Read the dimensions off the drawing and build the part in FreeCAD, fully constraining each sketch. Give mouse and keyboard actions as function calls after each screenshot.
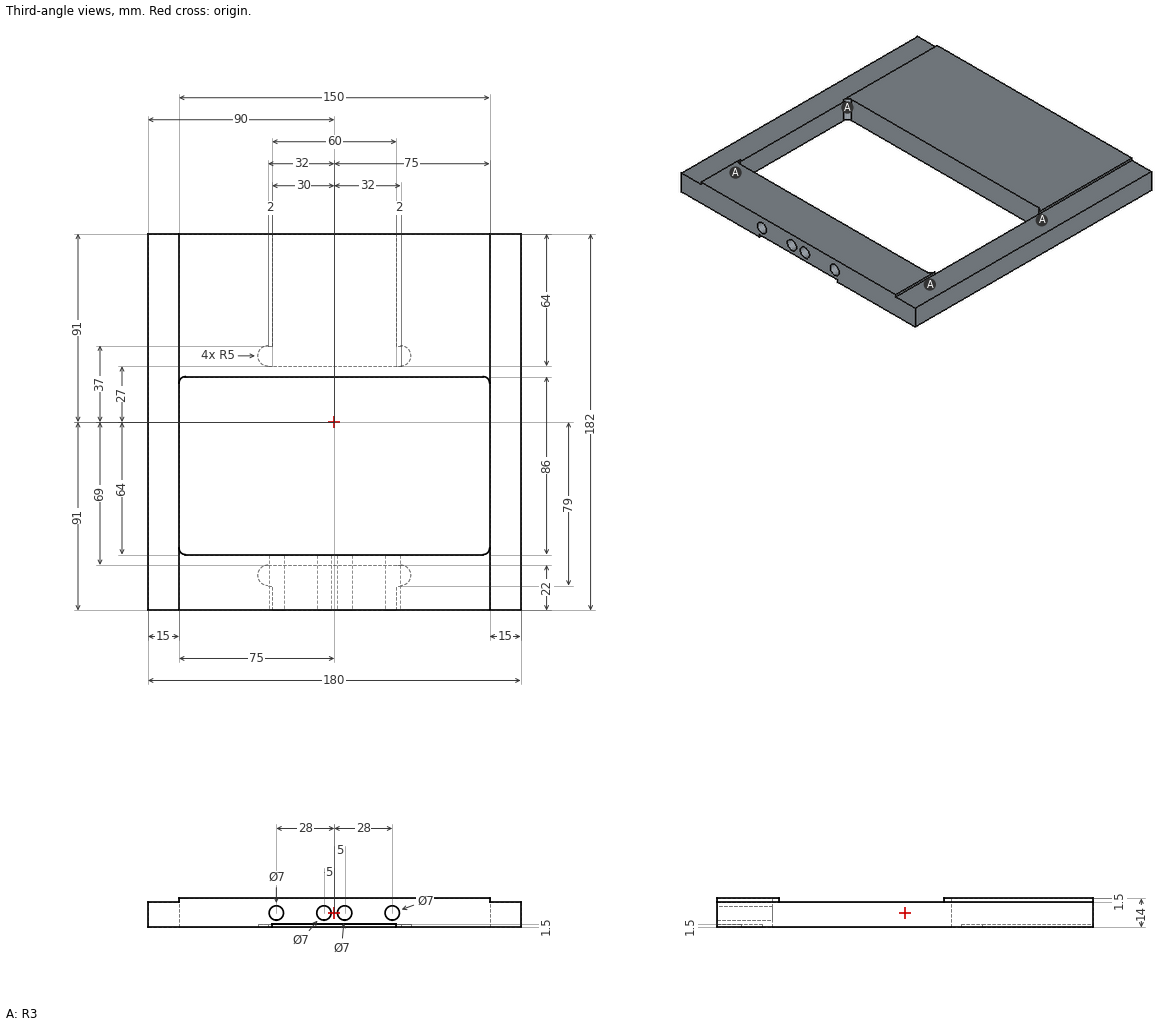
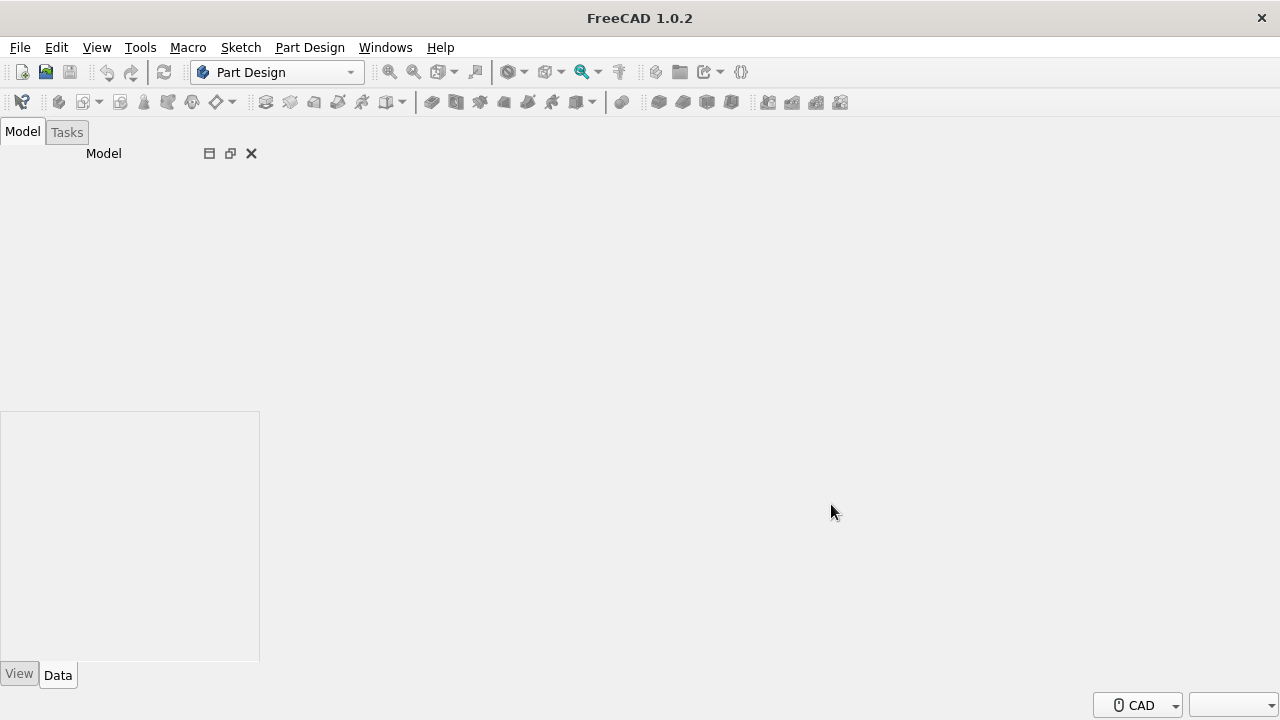
key(ctrl+n)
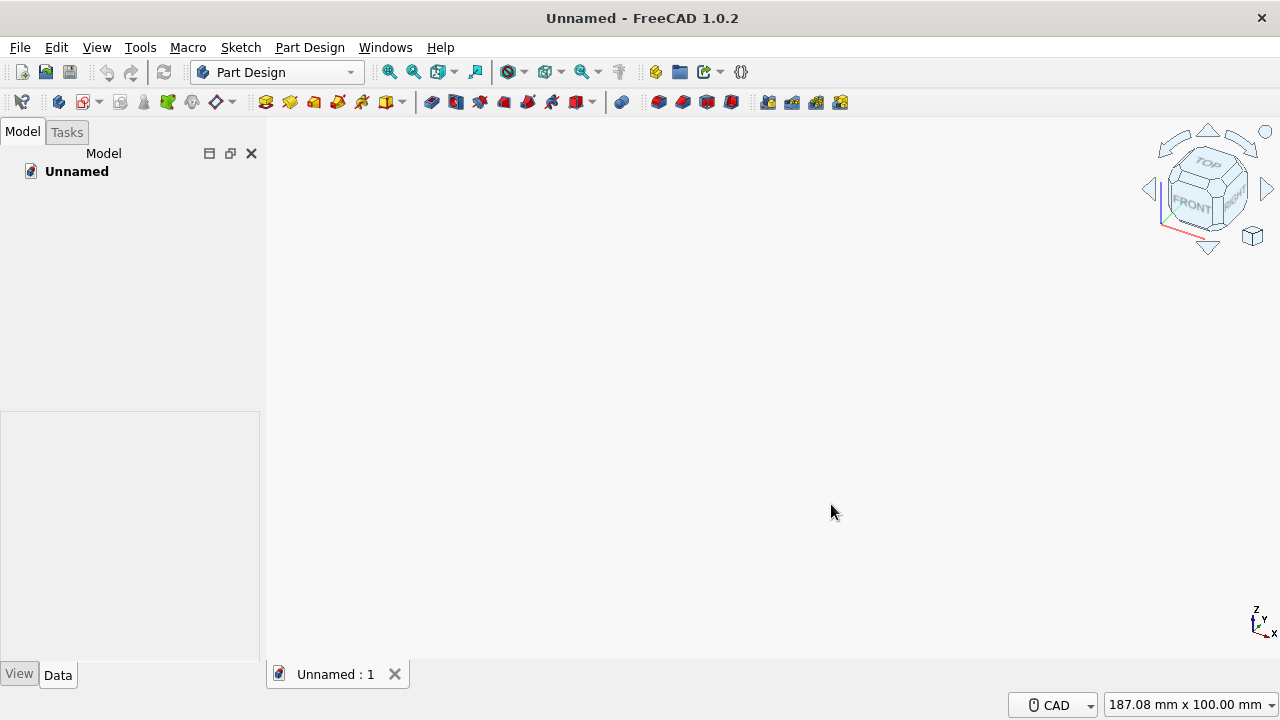
click(84, 102)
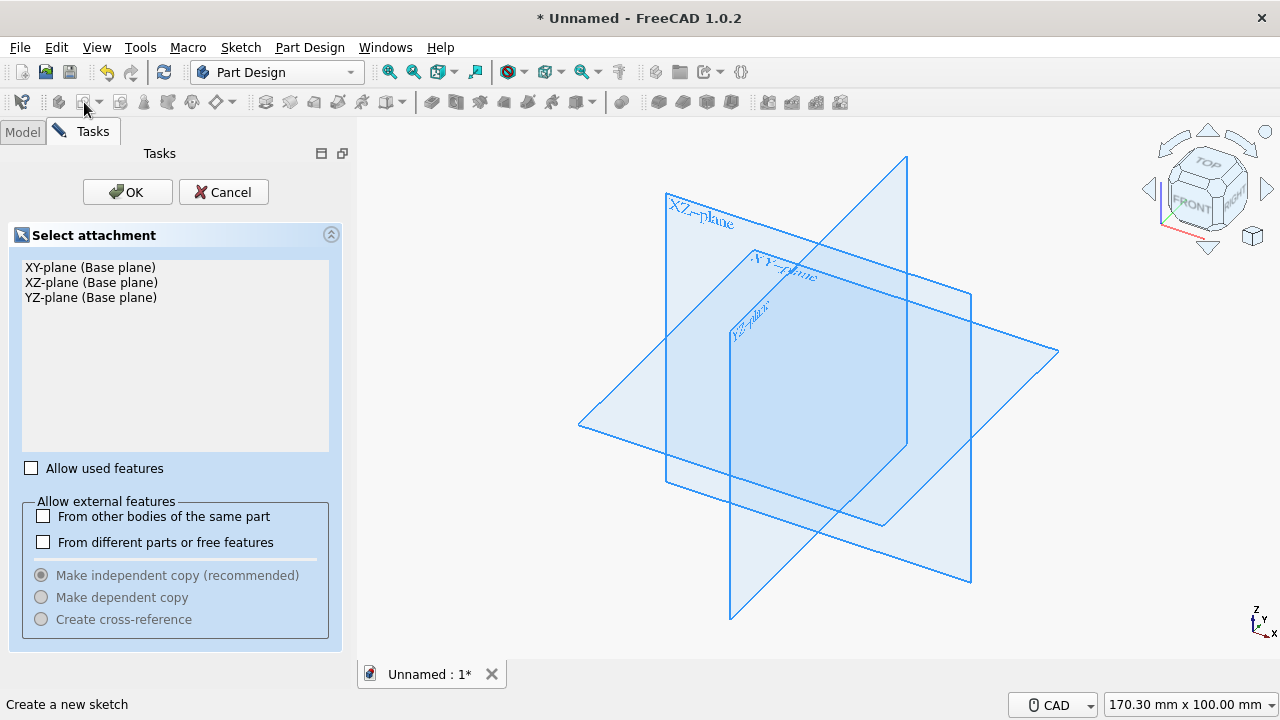
click(82, 268)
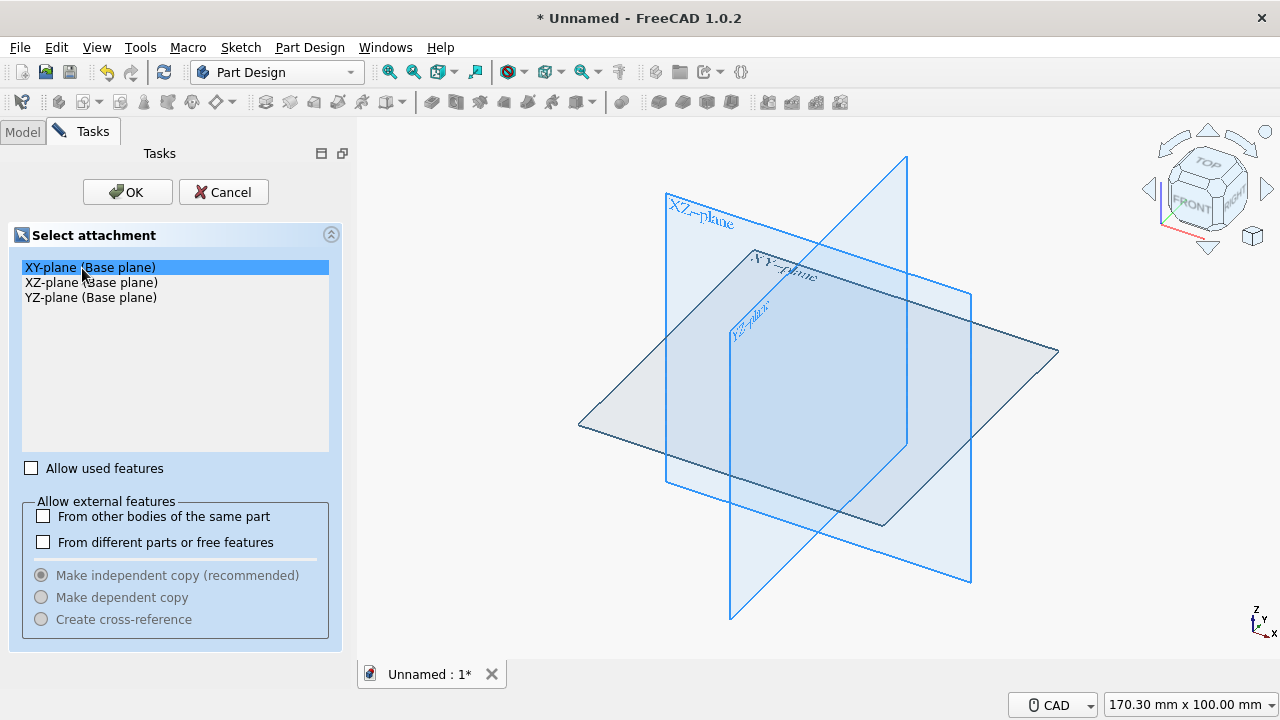
click(128, 192)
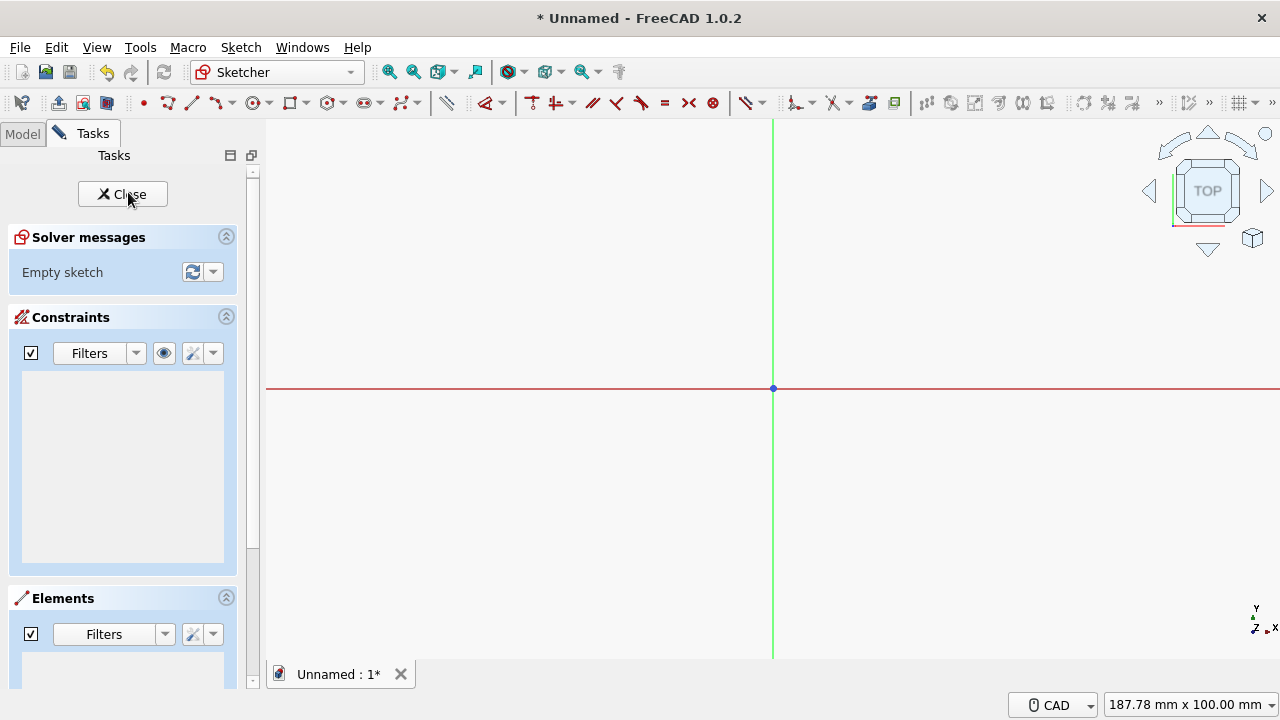
scroll(665, 389, down, 5)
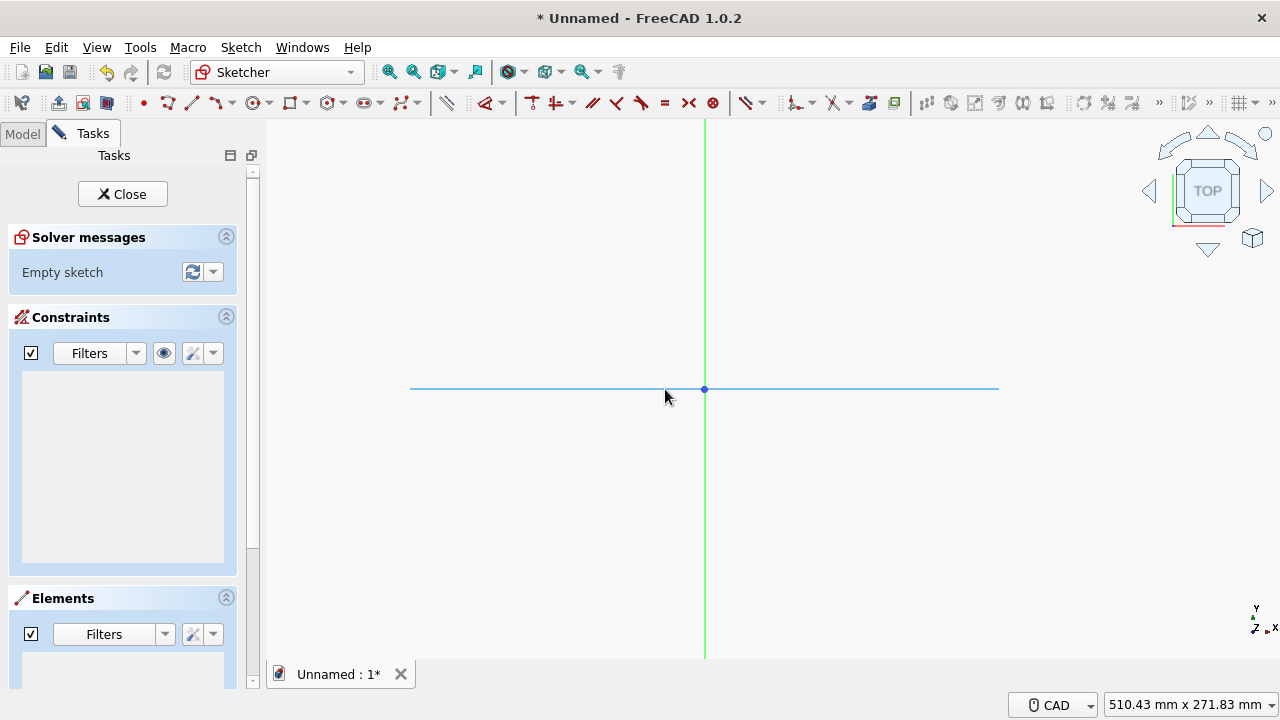
click(308, 104)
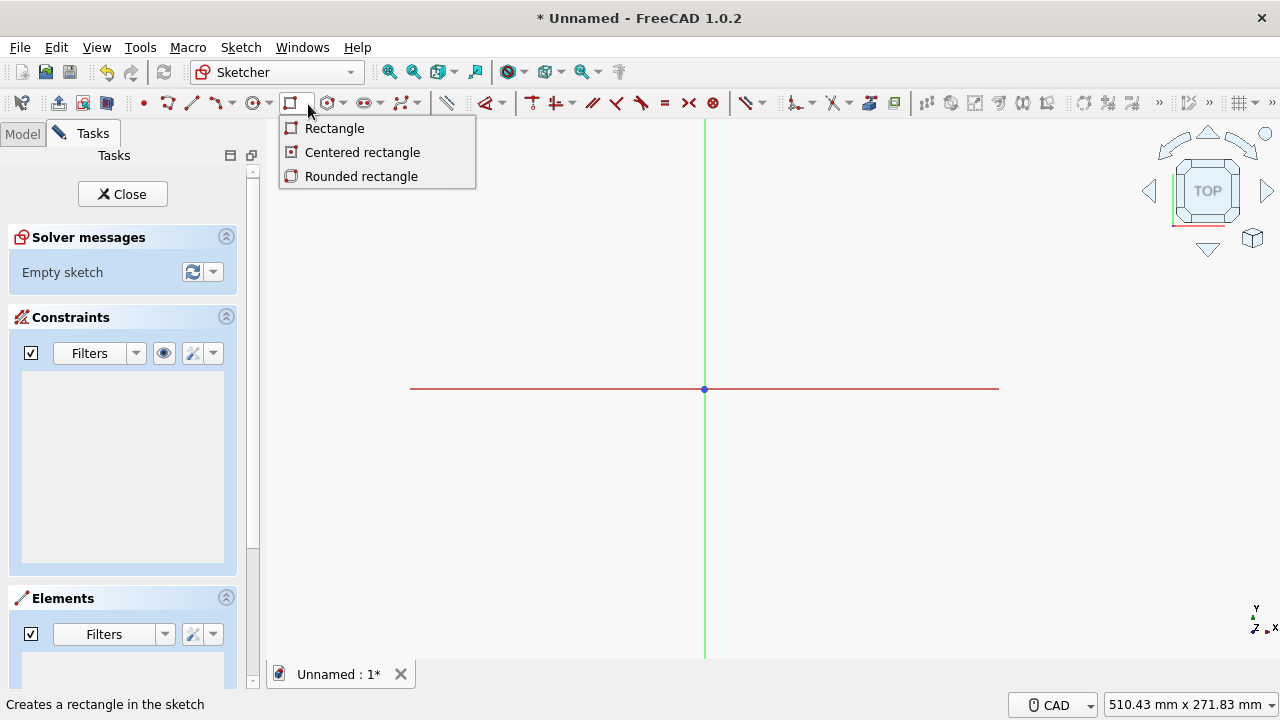
click(378, 152)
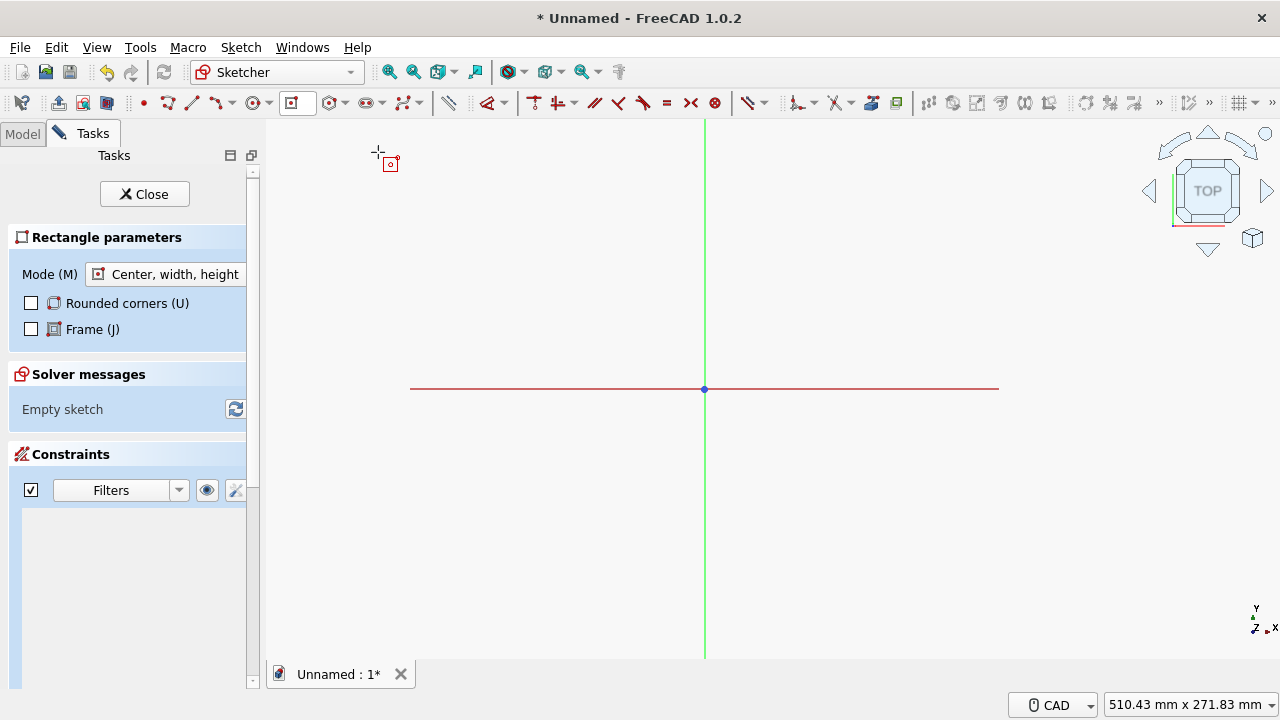
click(705, 389)
move(884, 209)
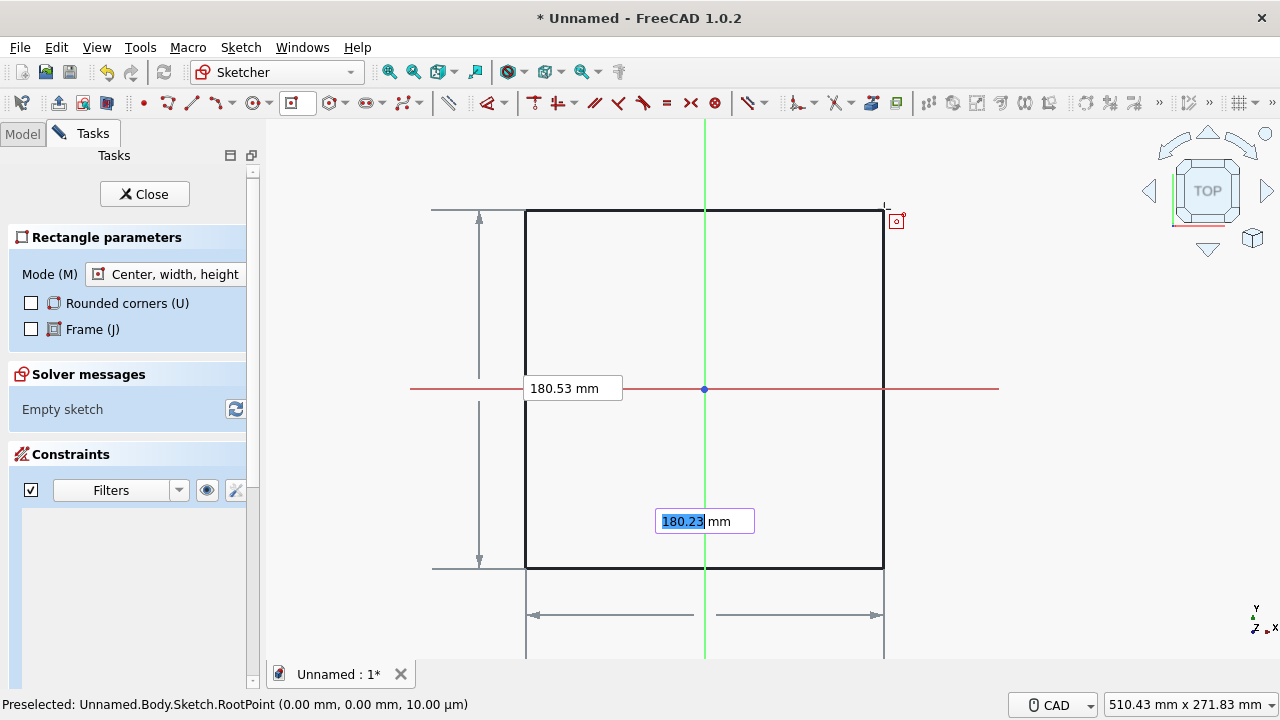
text(180)
key(Tab)
text(182)
key(Return)
key(Escape)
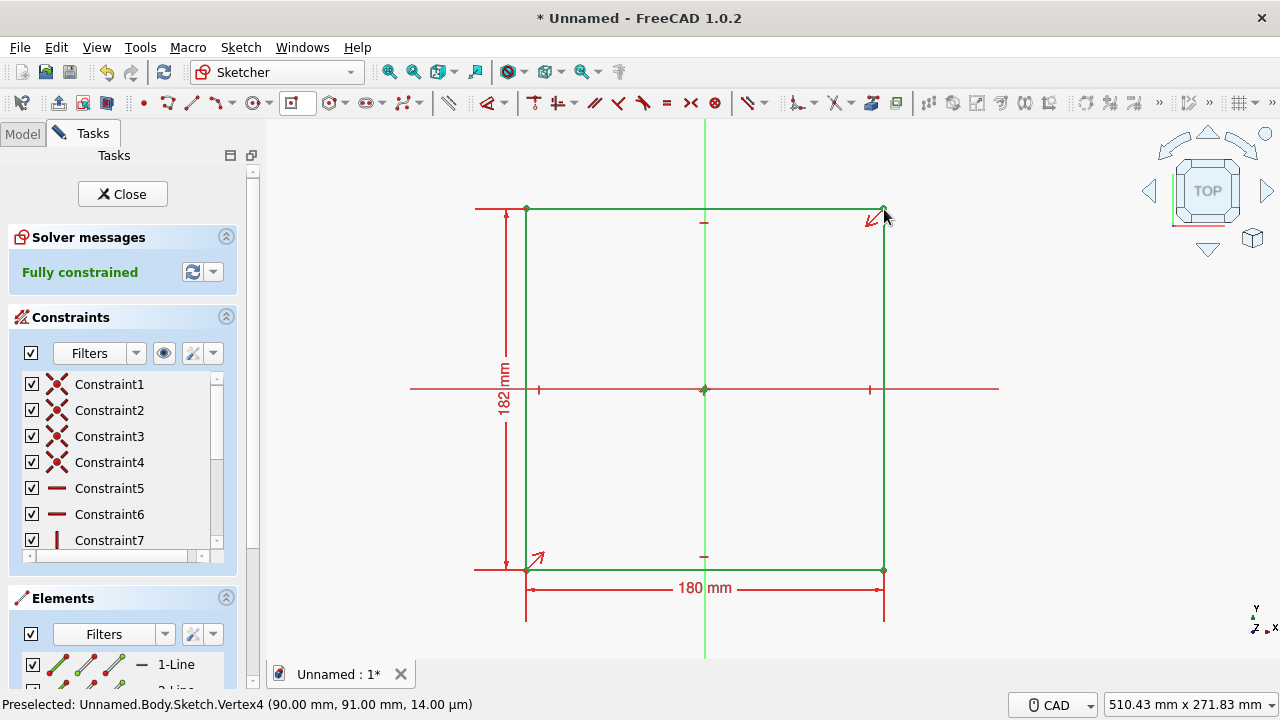
click(123, 194)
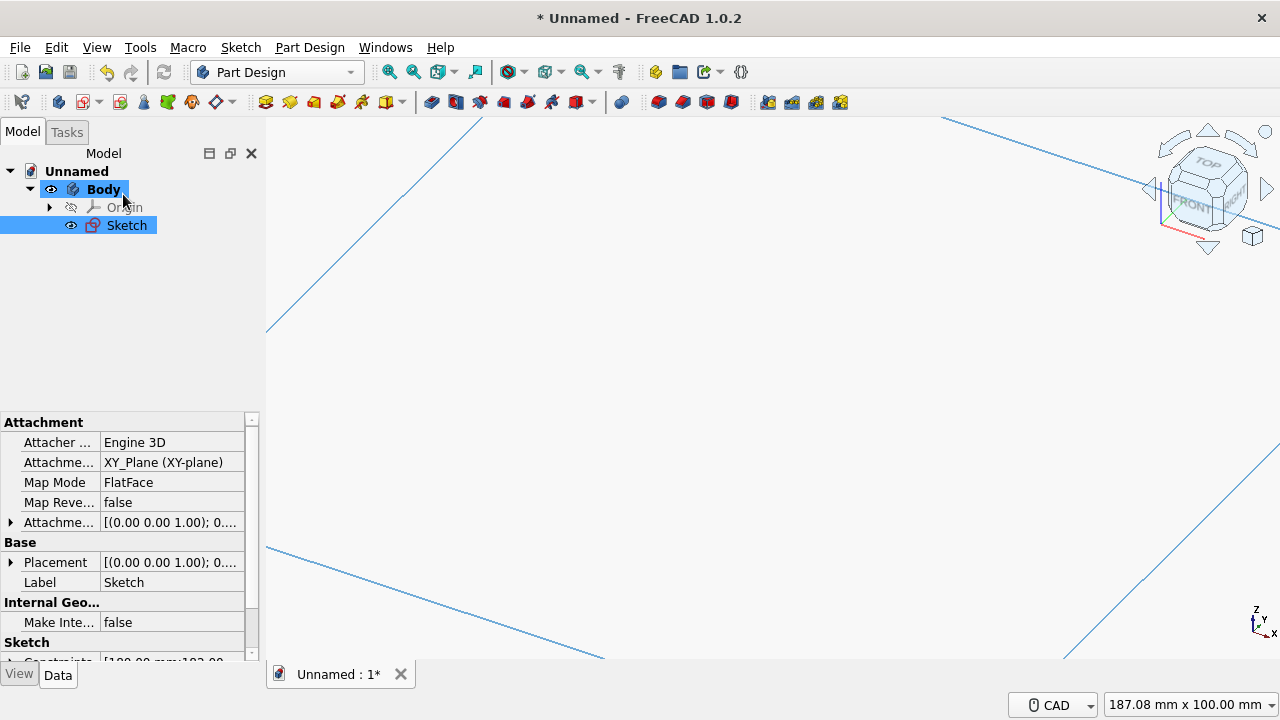
click(266, 102)